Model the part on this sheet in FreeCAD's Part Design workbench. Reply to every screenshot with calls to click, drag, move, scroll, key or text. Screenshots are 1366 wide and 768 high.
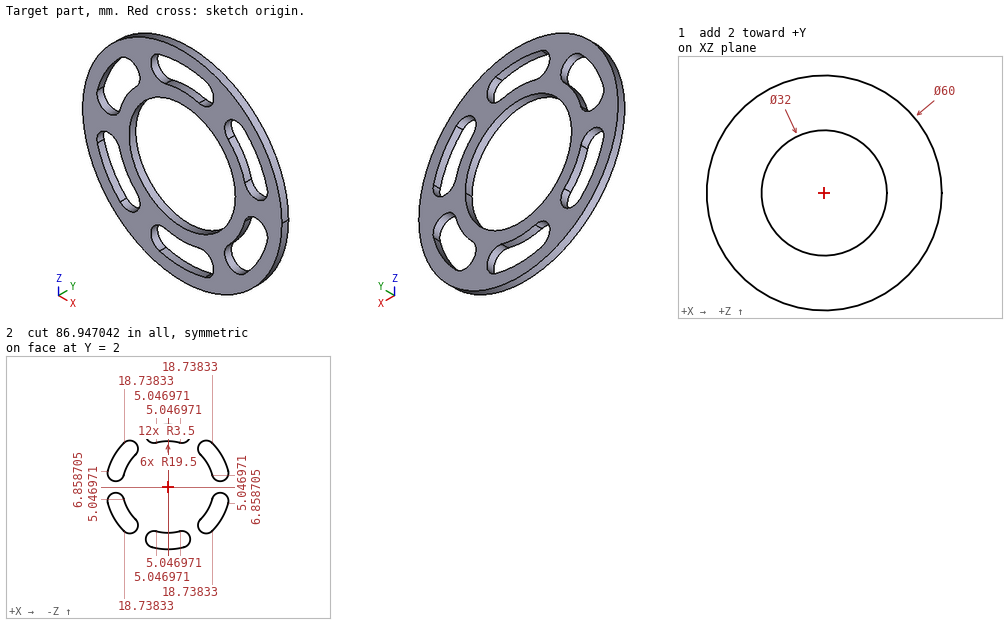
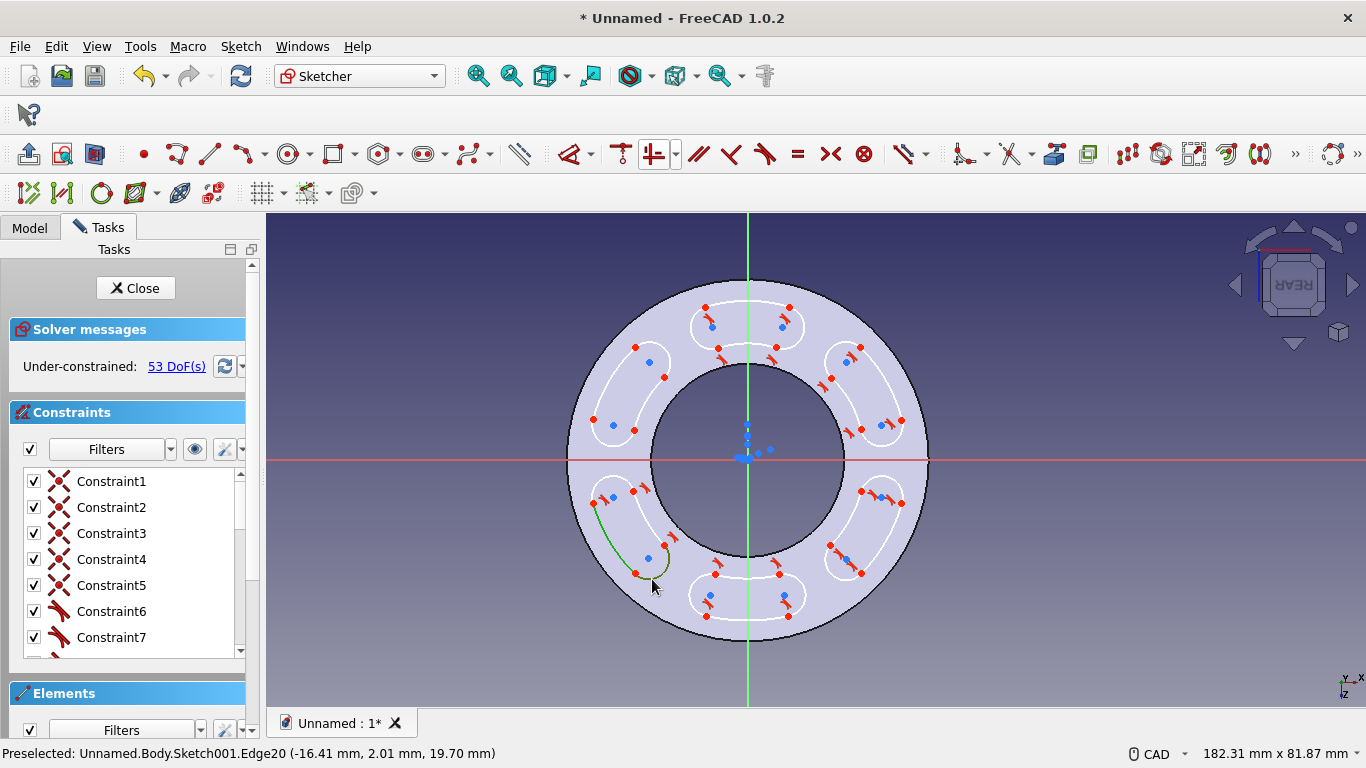
click(765, 154)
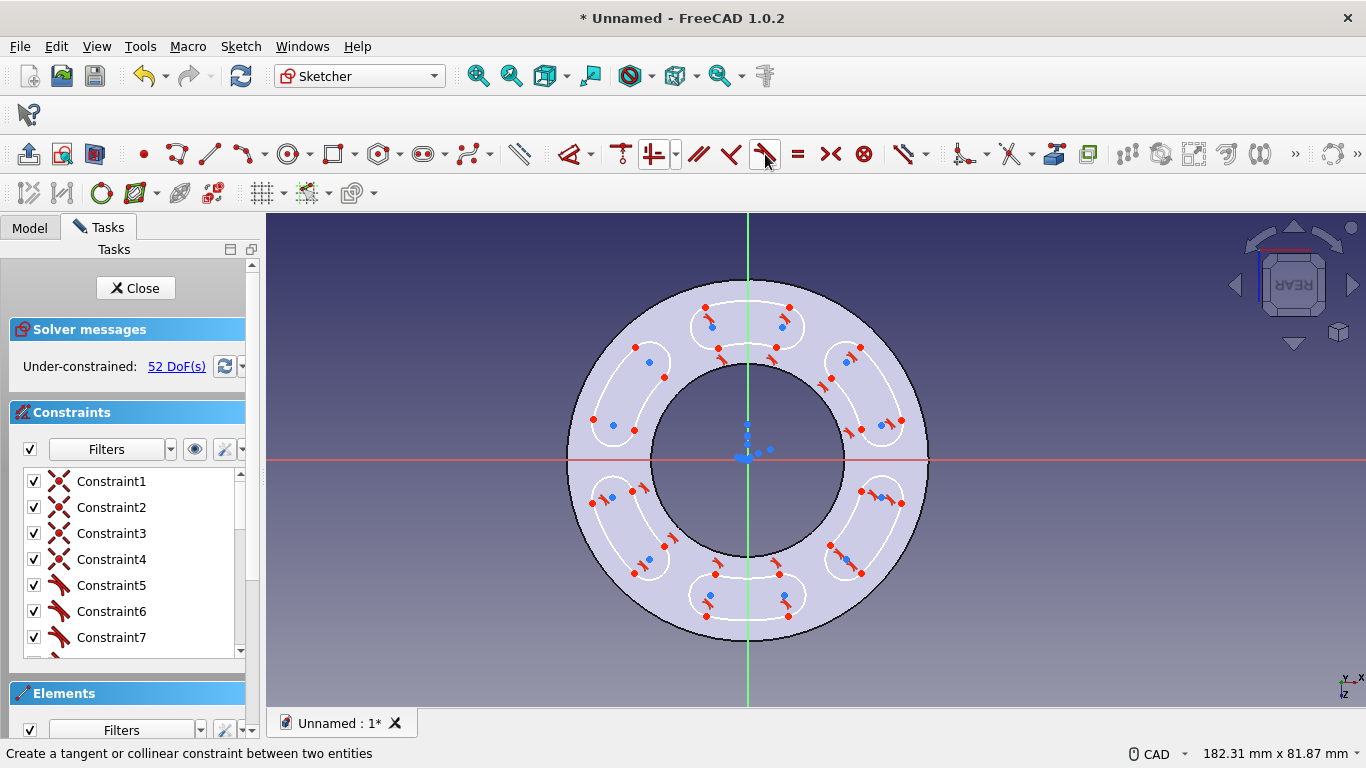
click(670, 360)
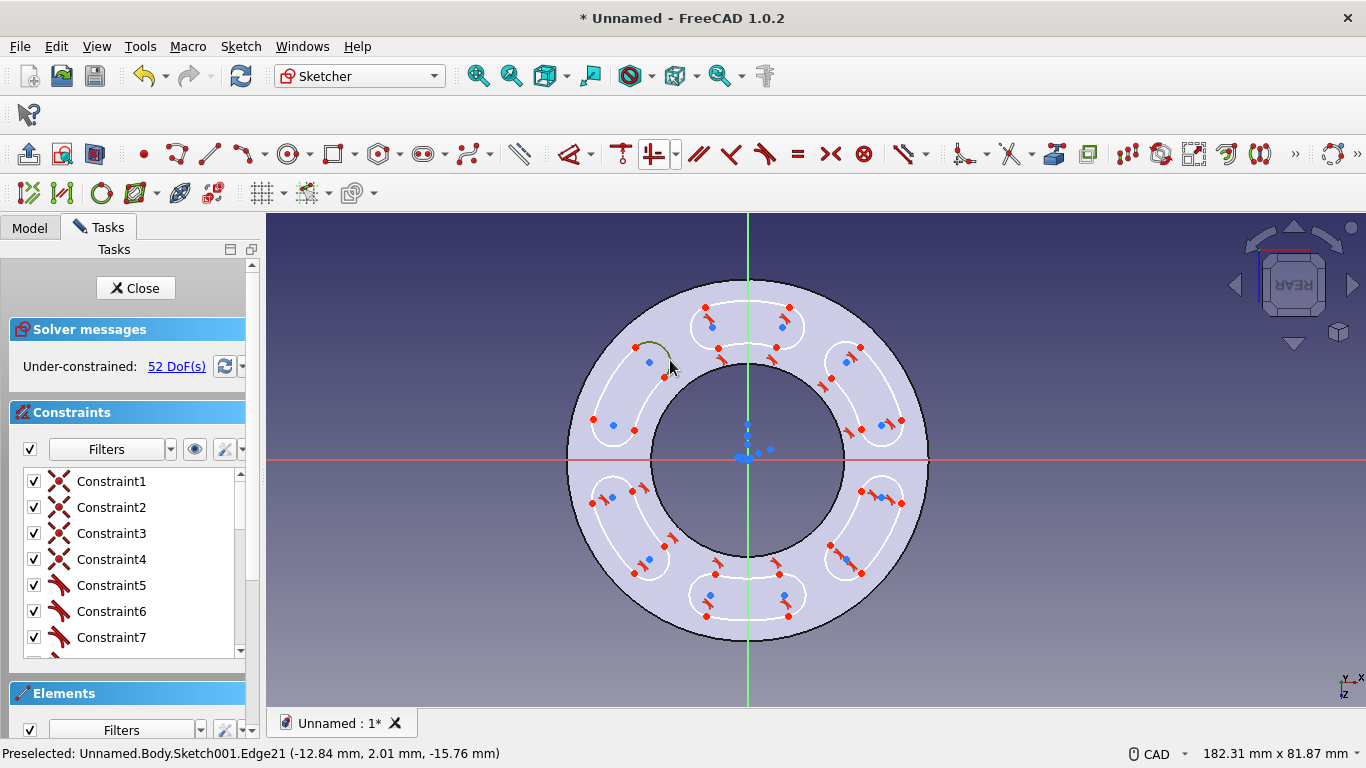
click(618, 367)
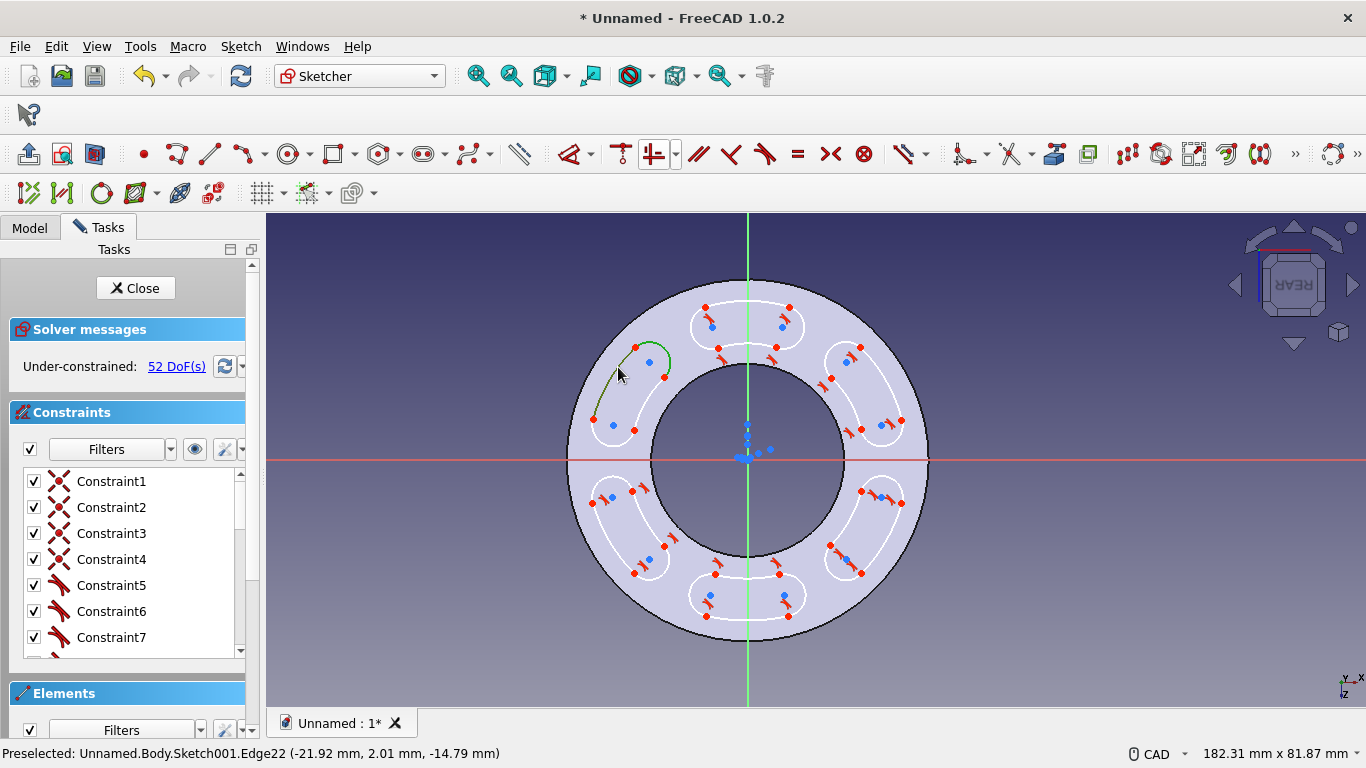
key(t)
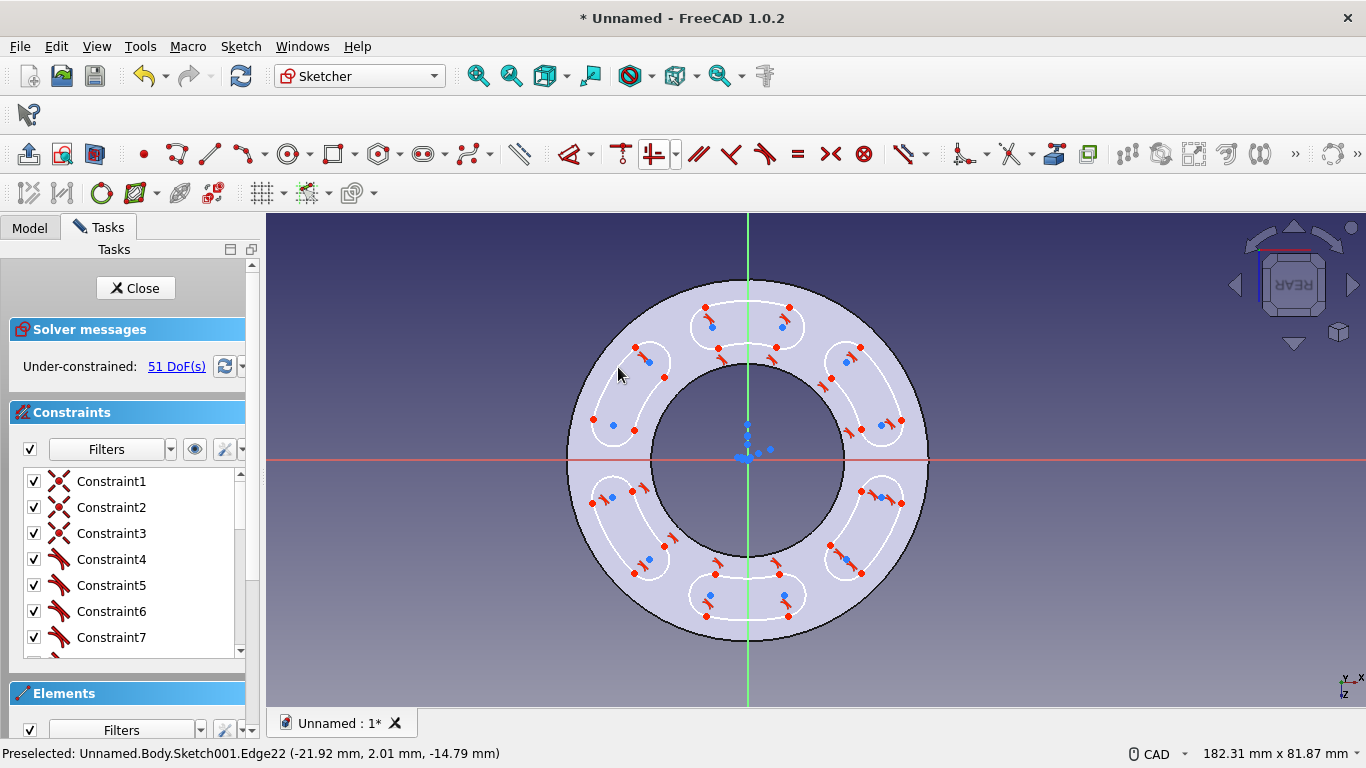
click(670, 360)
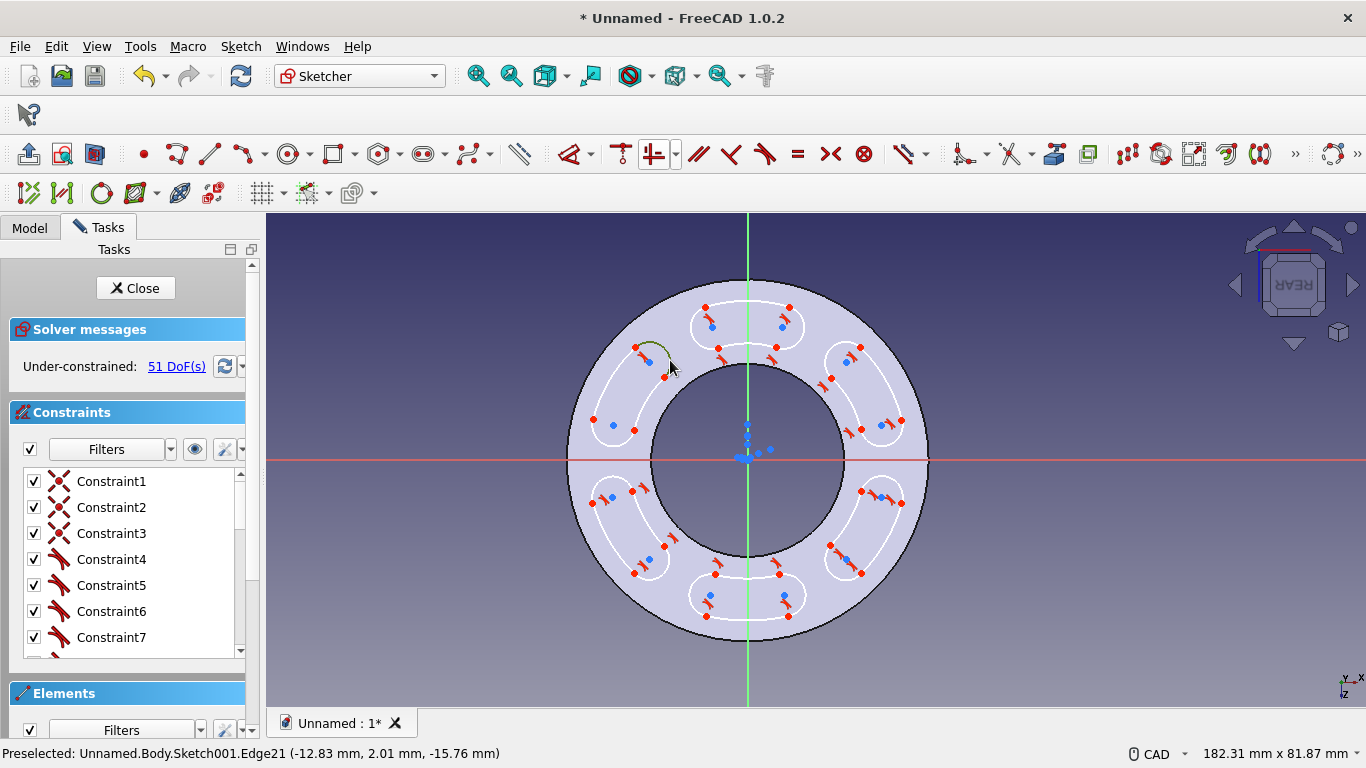
click(652, 392)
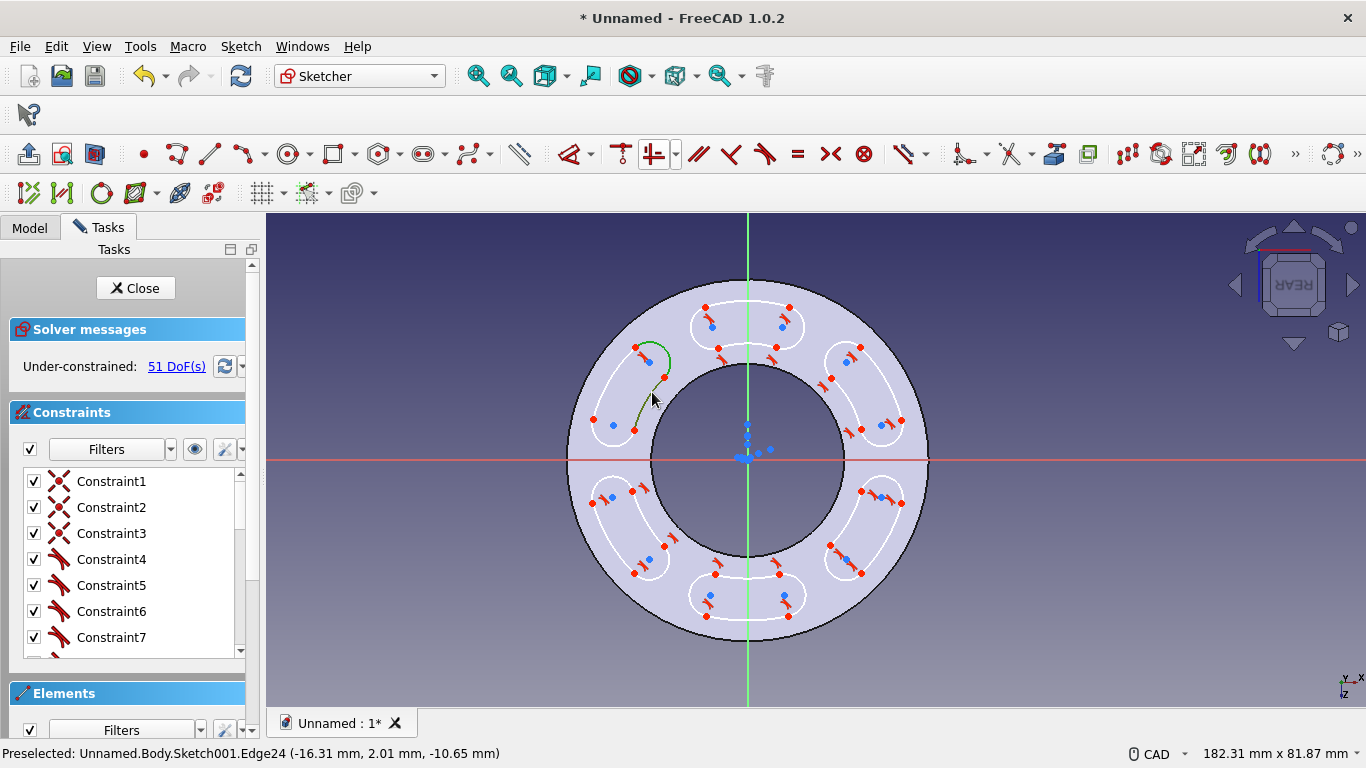
click(765, 154)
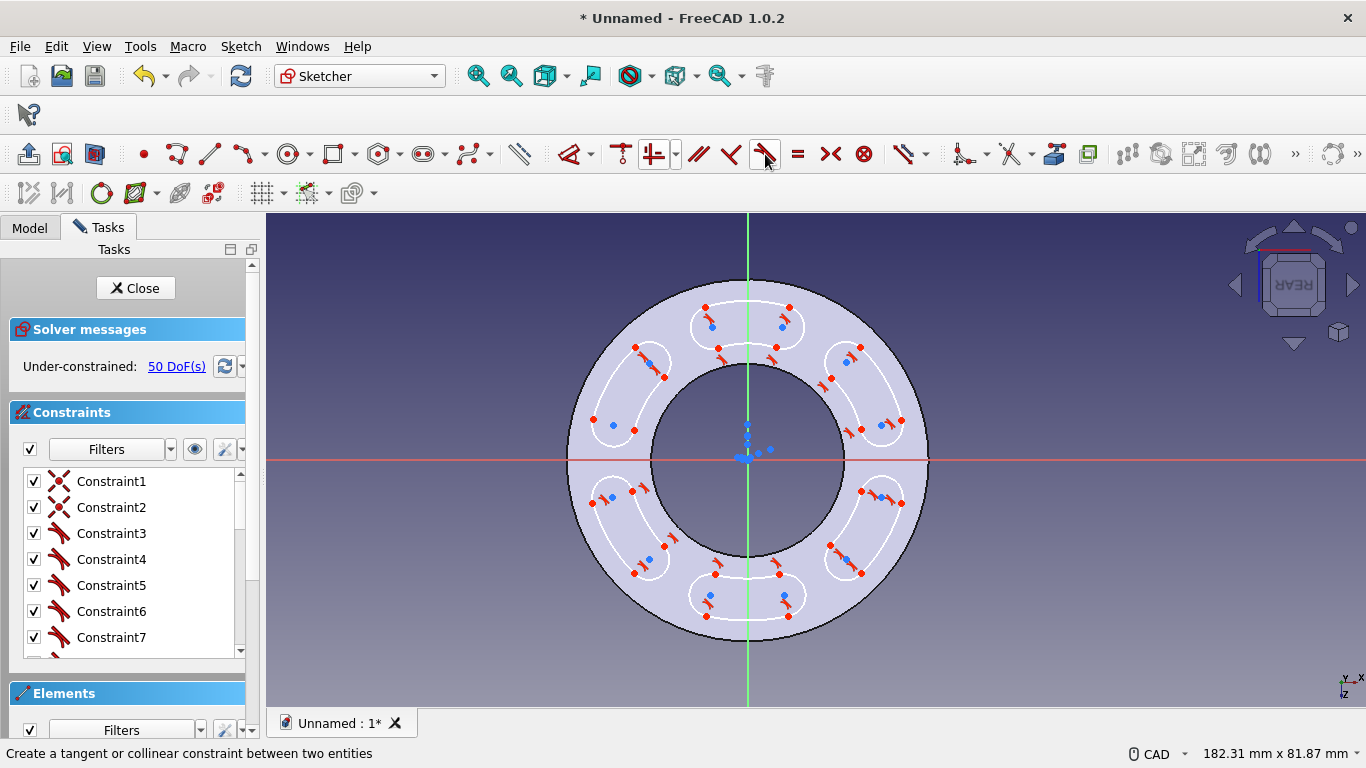
click(618, 367)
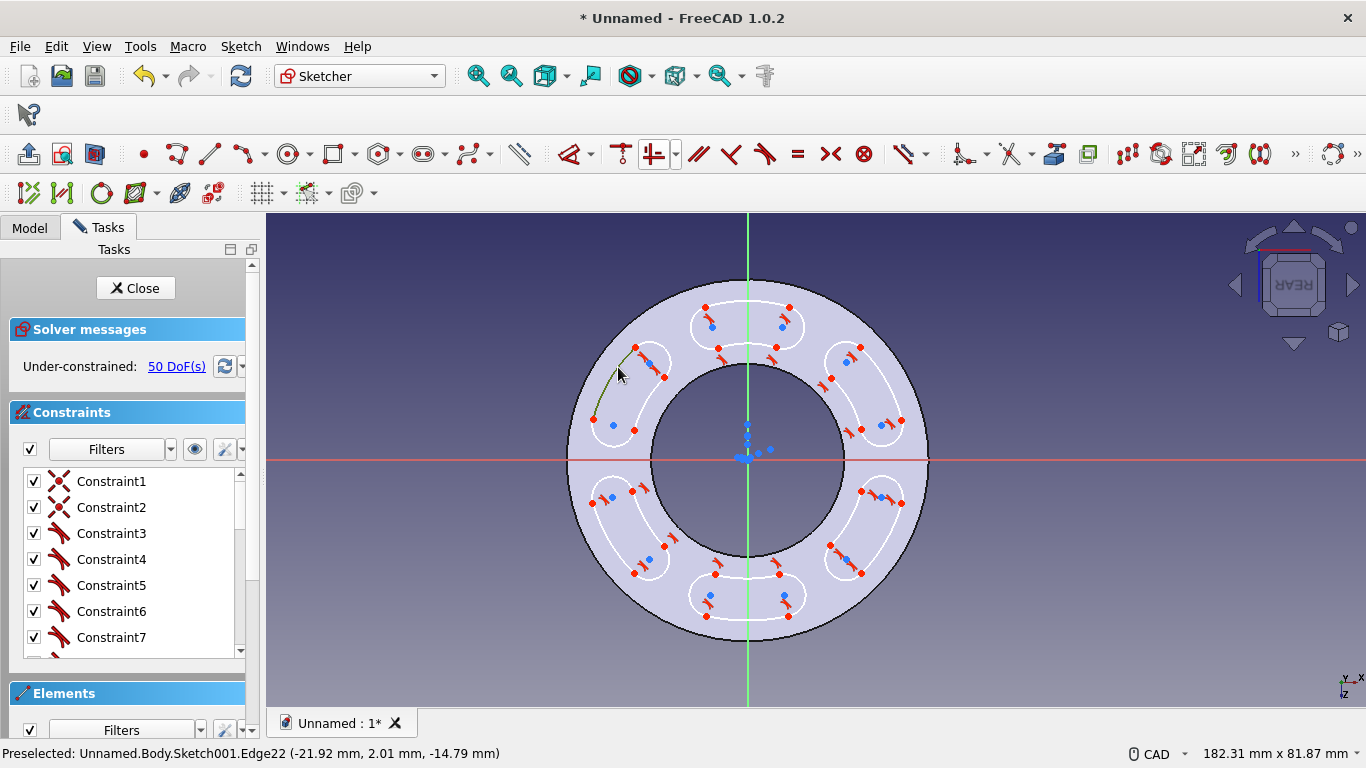
click(597, 439)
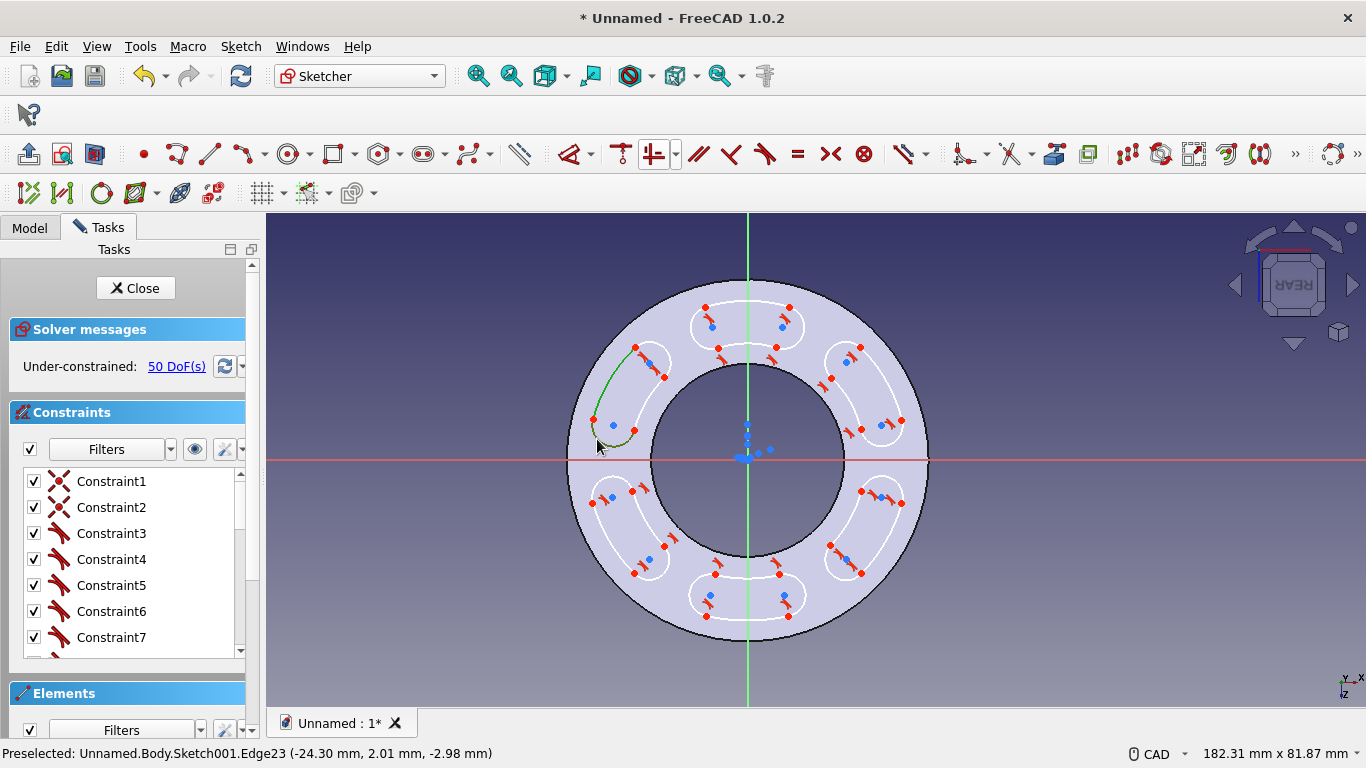
click(765, 154)